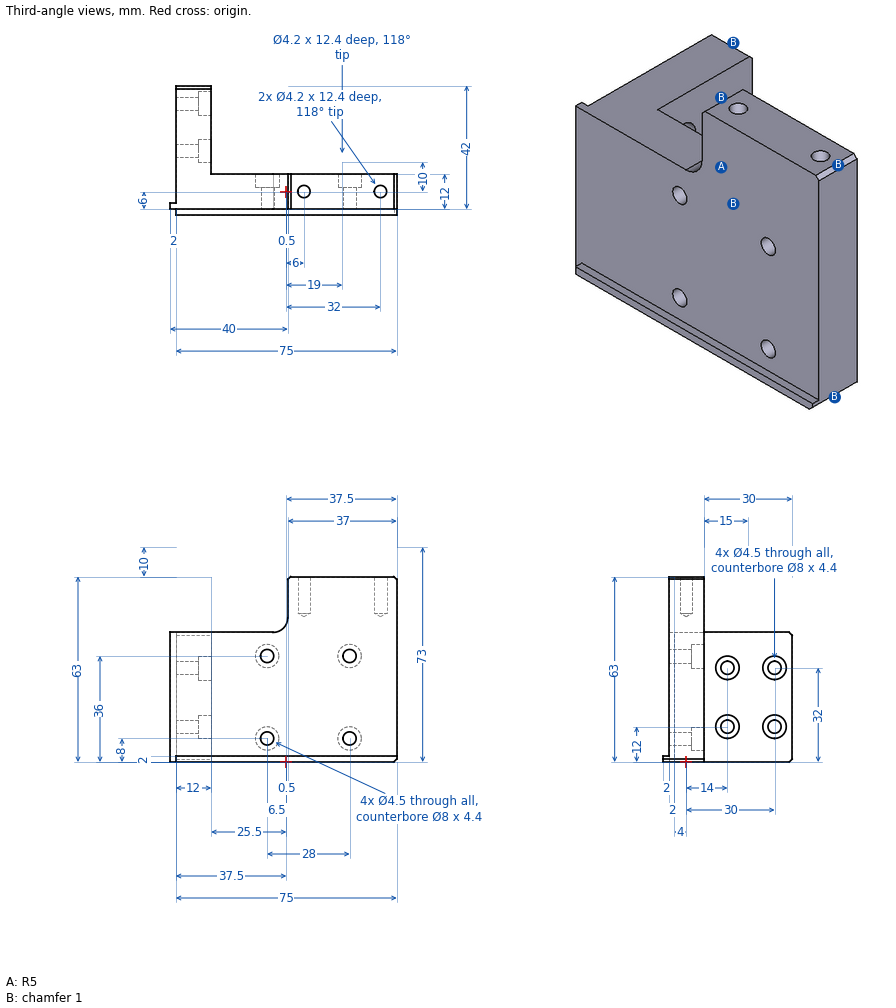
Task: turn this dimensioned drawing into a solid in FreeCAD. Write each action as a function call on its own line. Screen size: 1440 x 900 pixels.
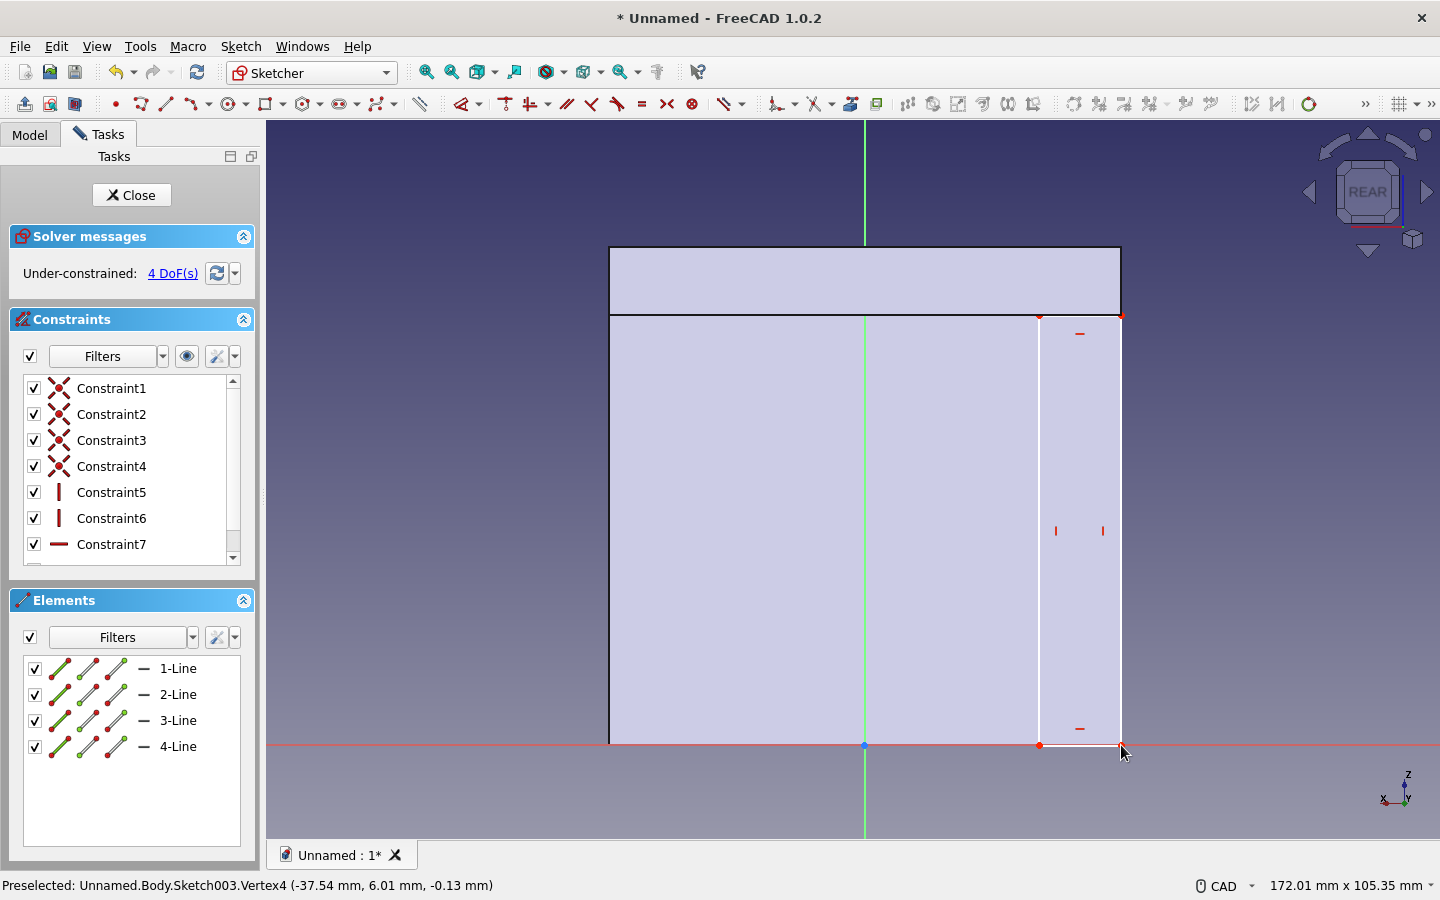
click(1039, 746)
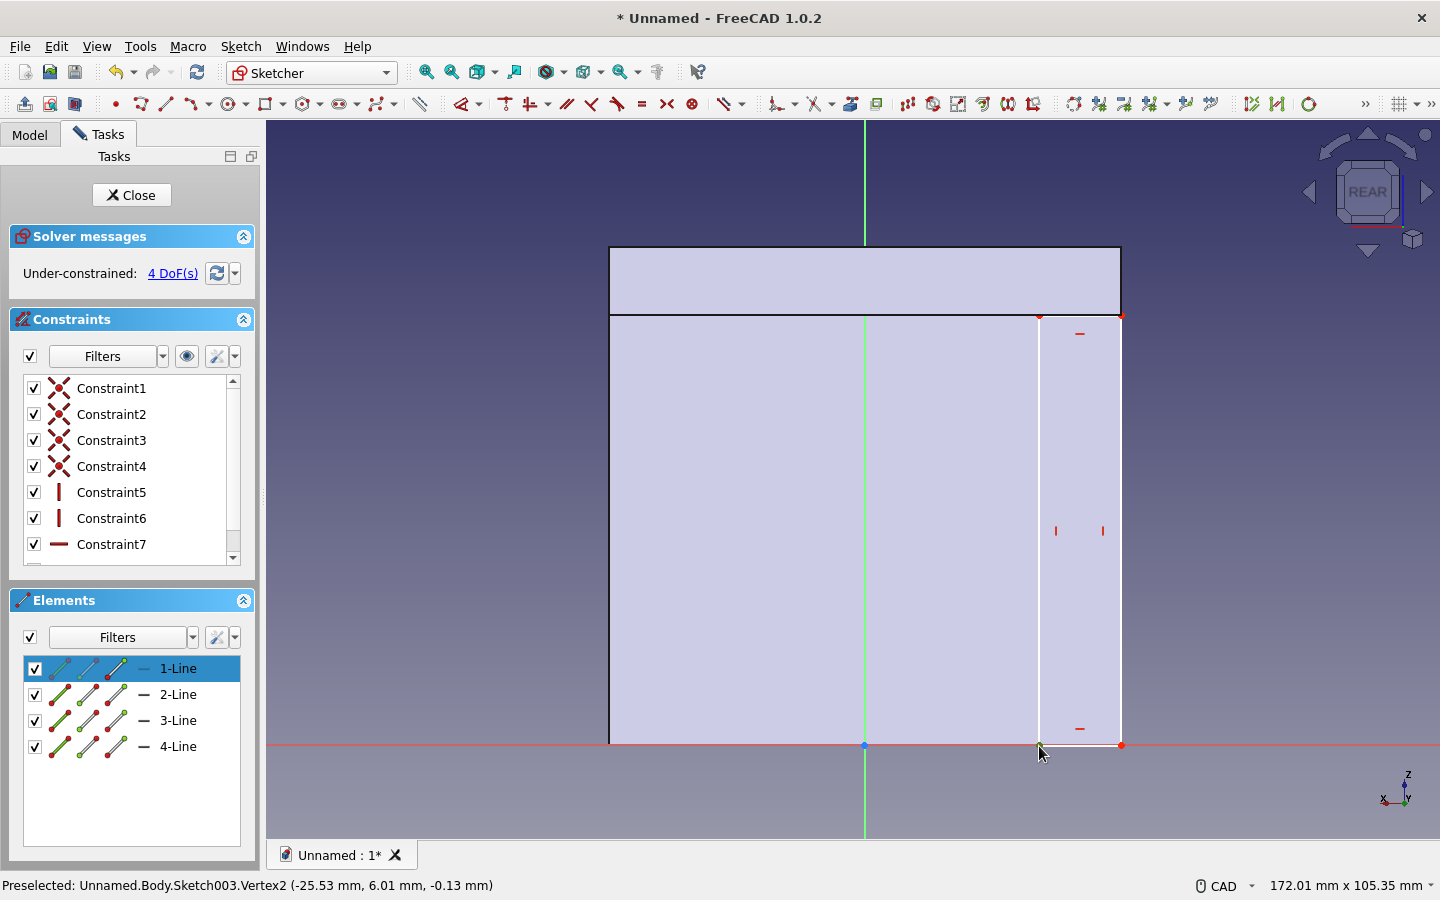
click(364, 745)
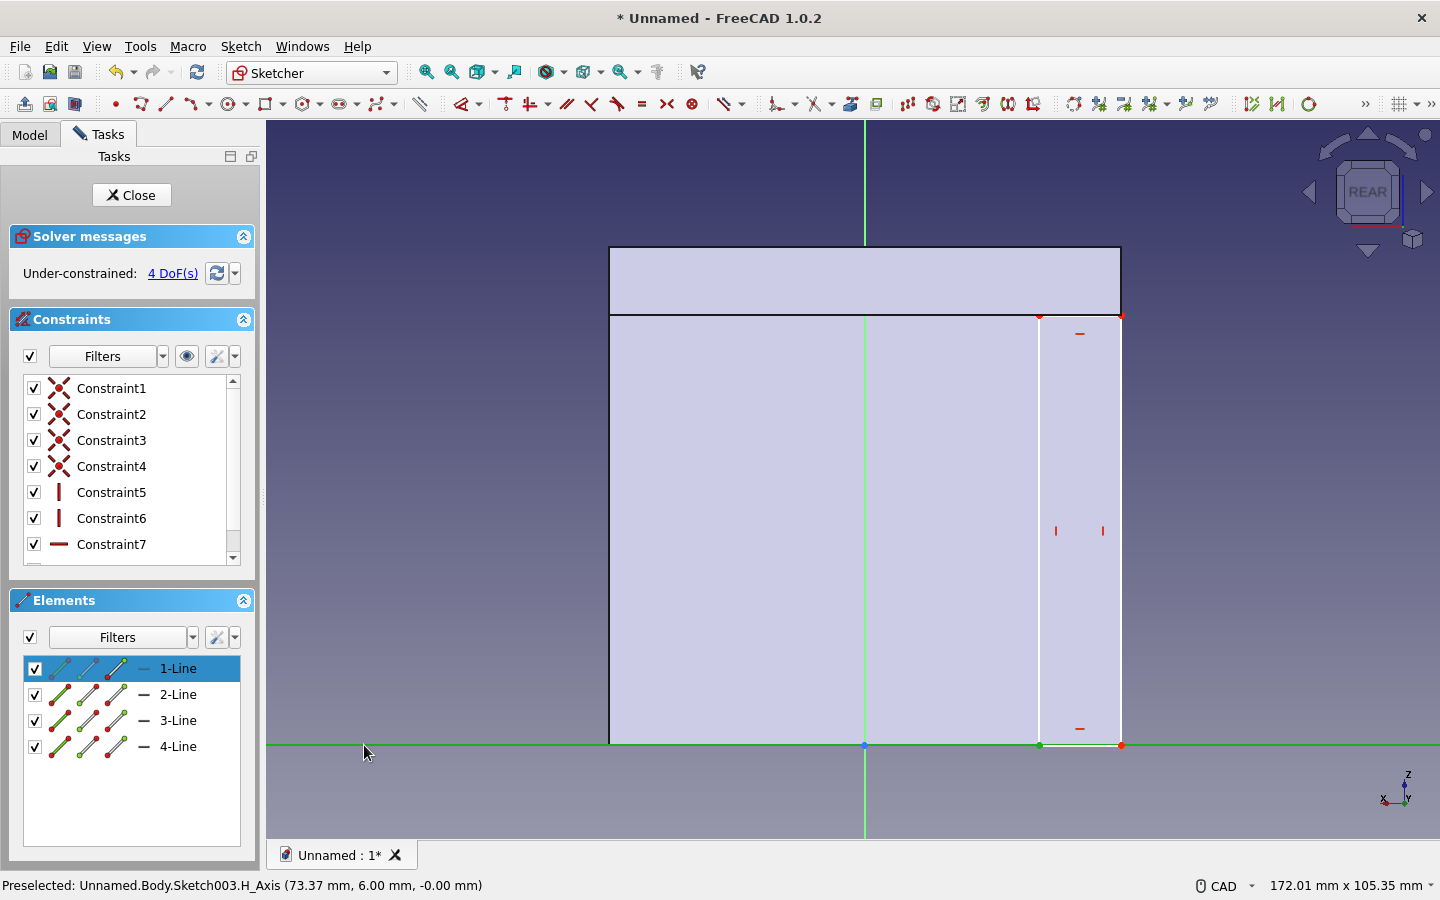
click(505, 104)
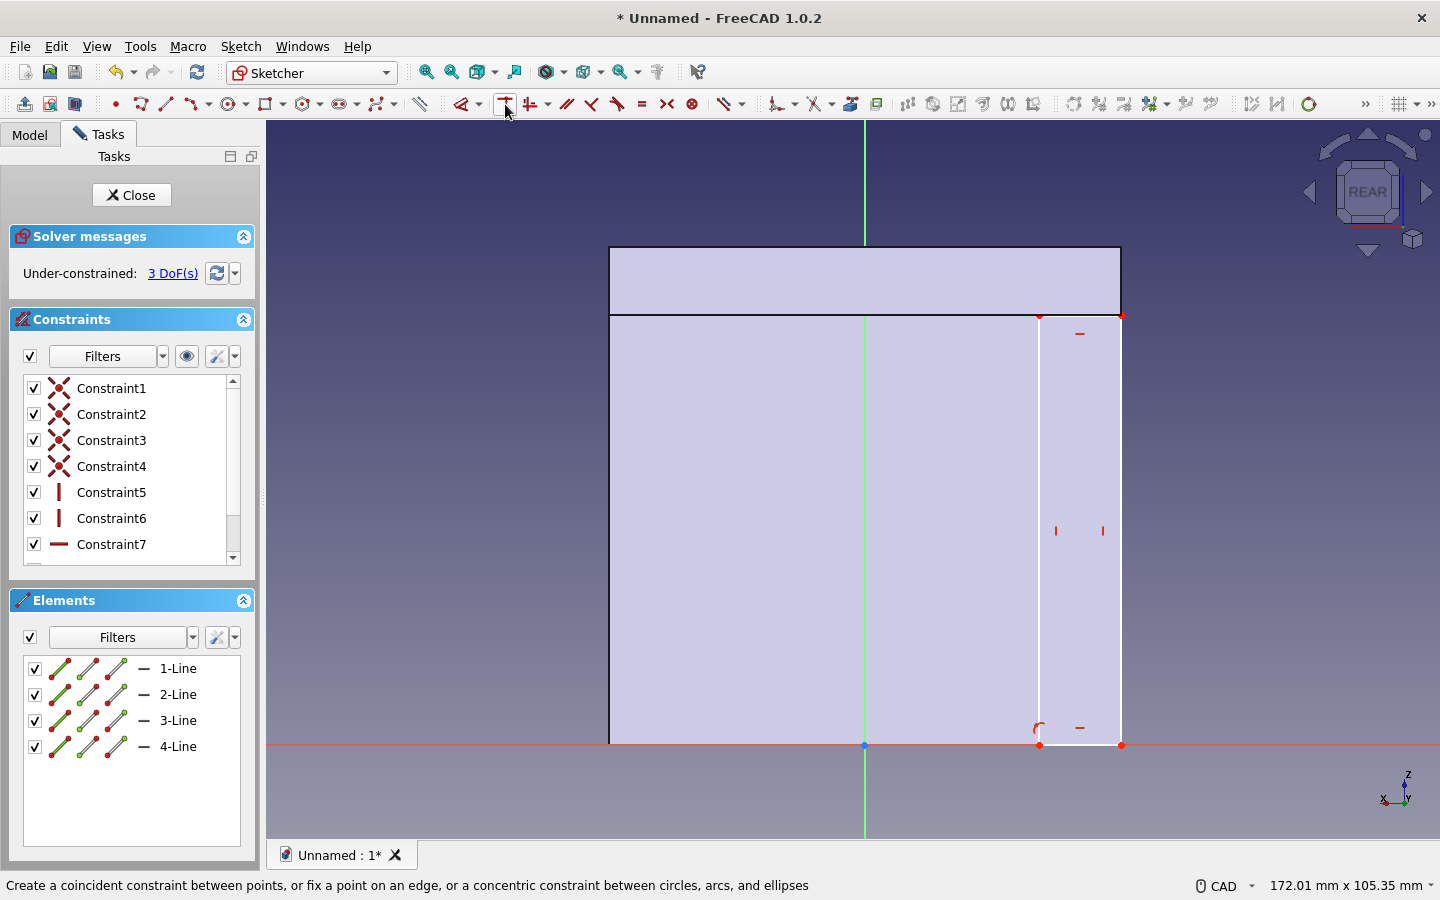
click(460, 104)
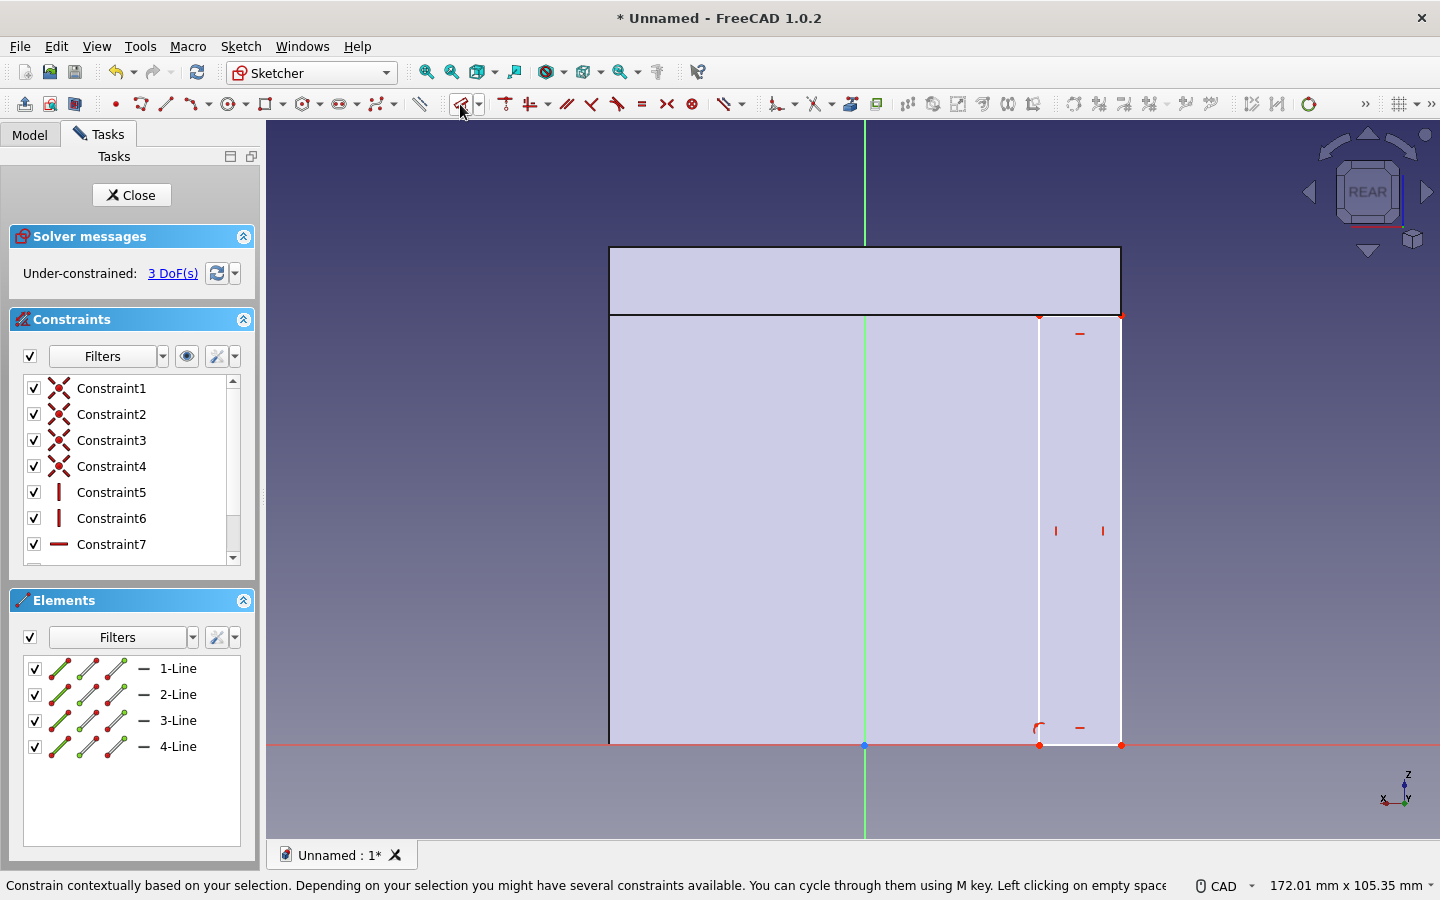
click(1039, 445)
click(1073, 531)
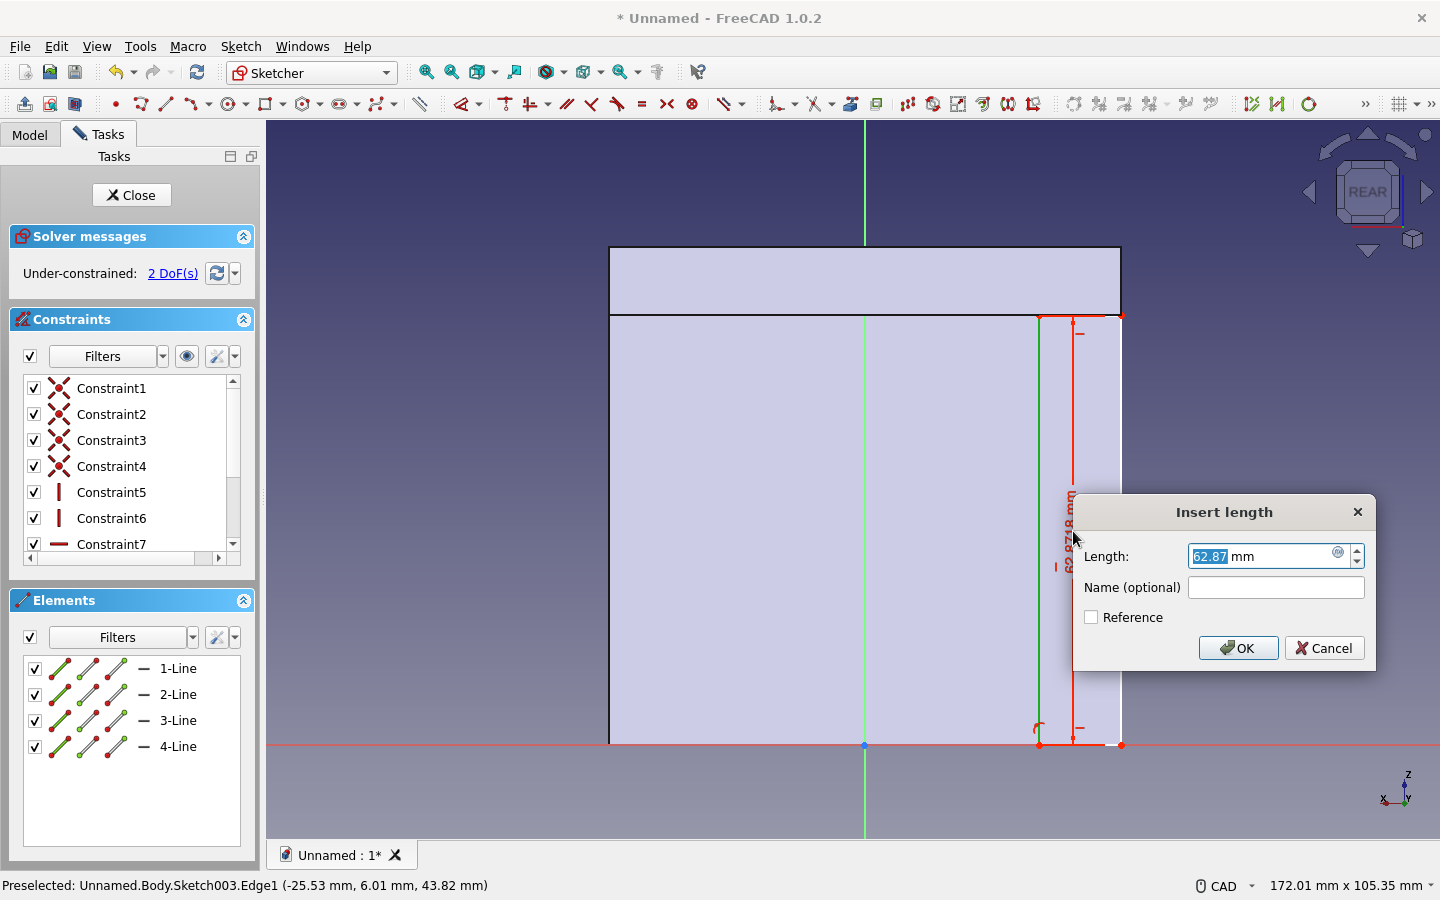
text(63)
key(Return)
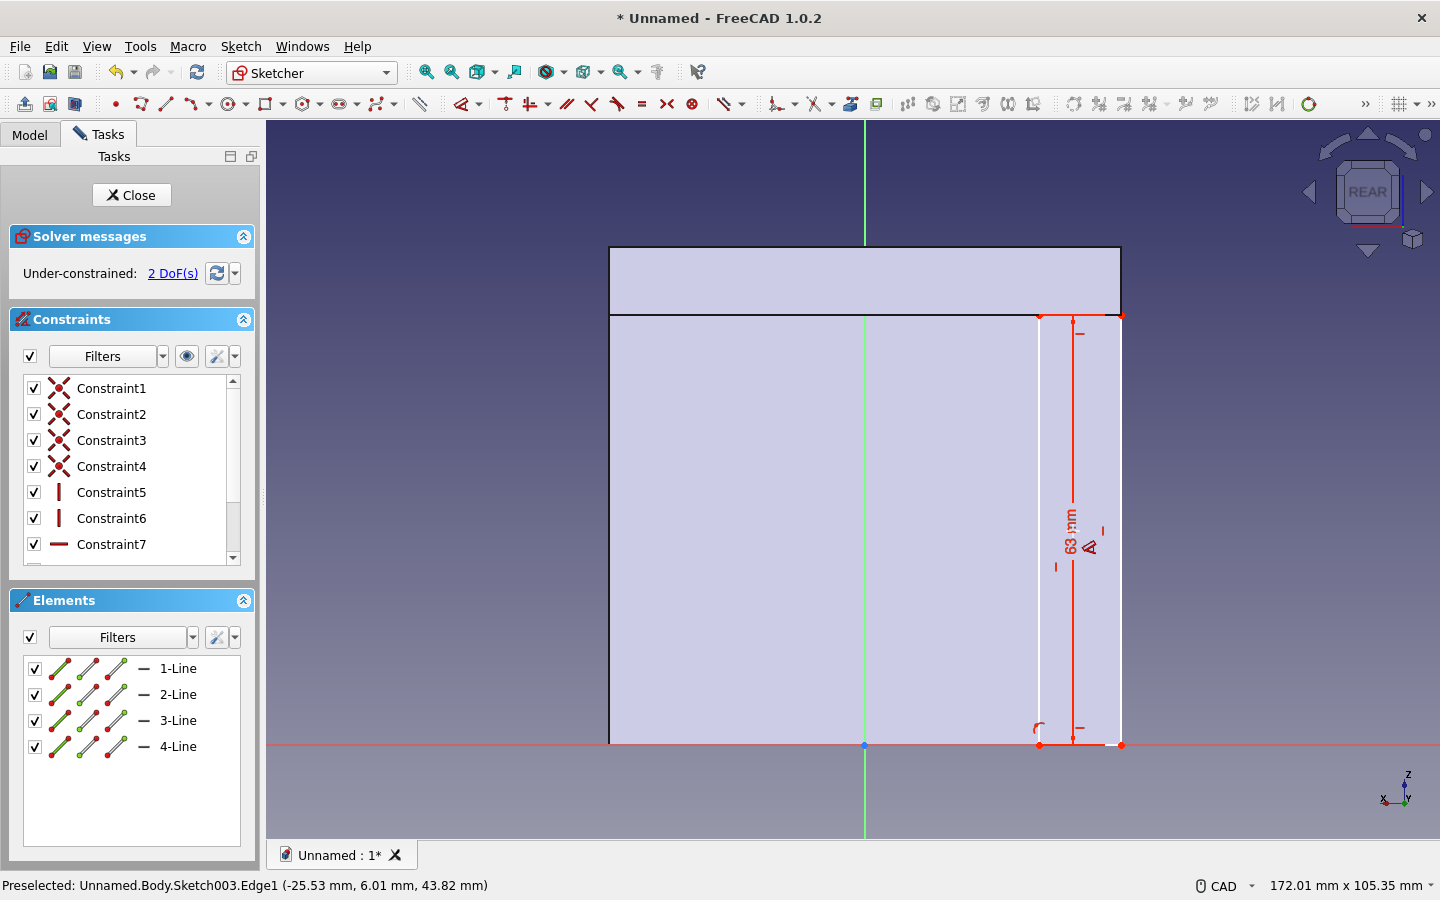
click(1064, 745)
click(1080, 779)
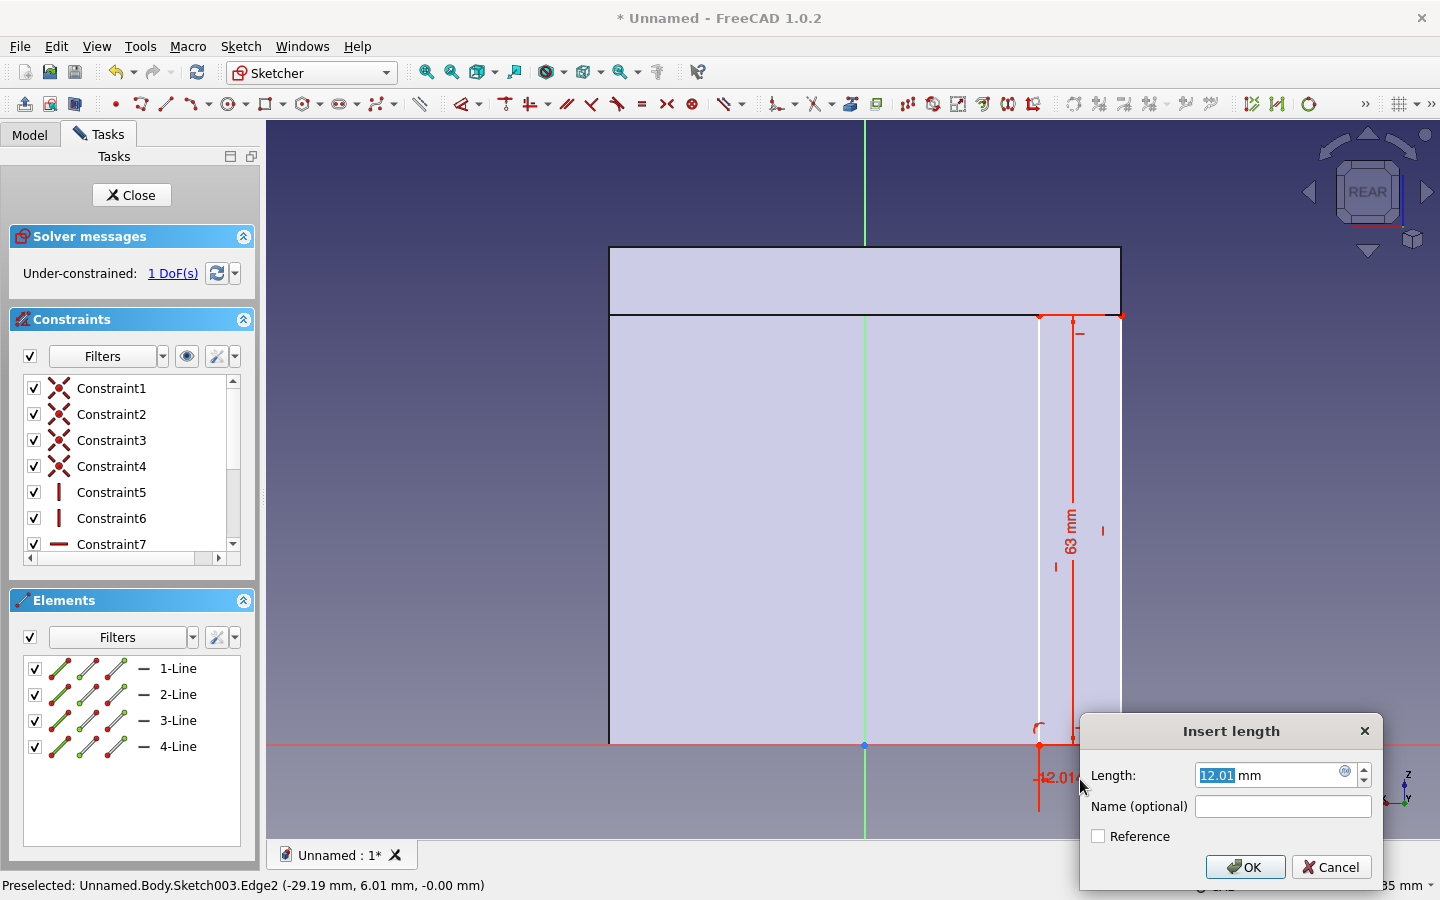
text(12)
key(Return)